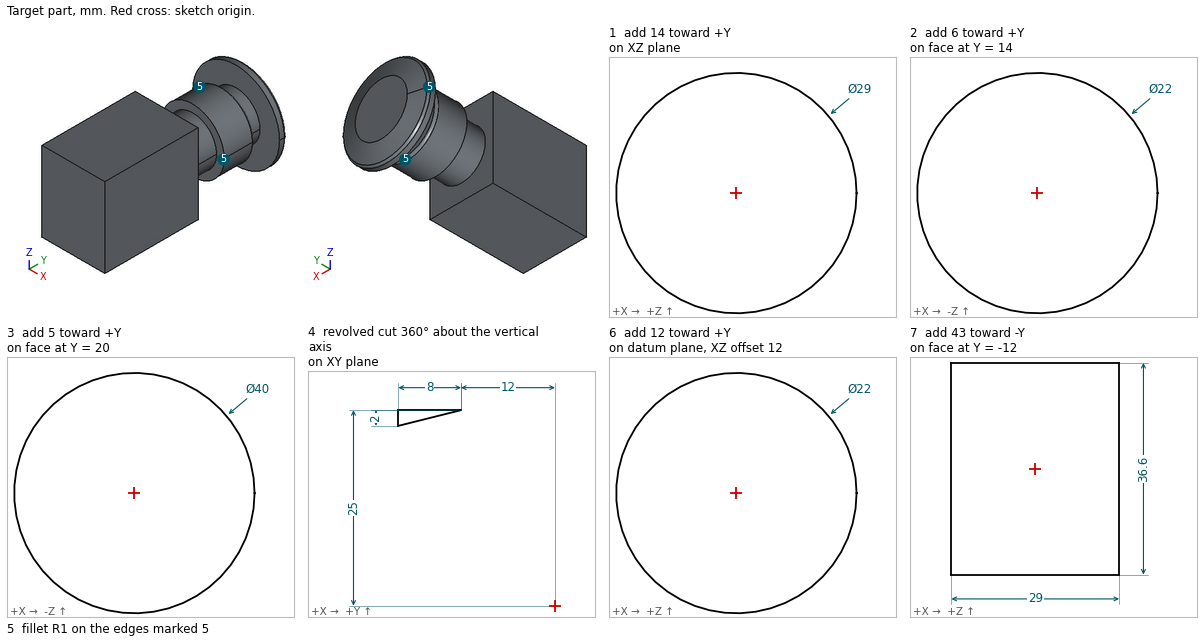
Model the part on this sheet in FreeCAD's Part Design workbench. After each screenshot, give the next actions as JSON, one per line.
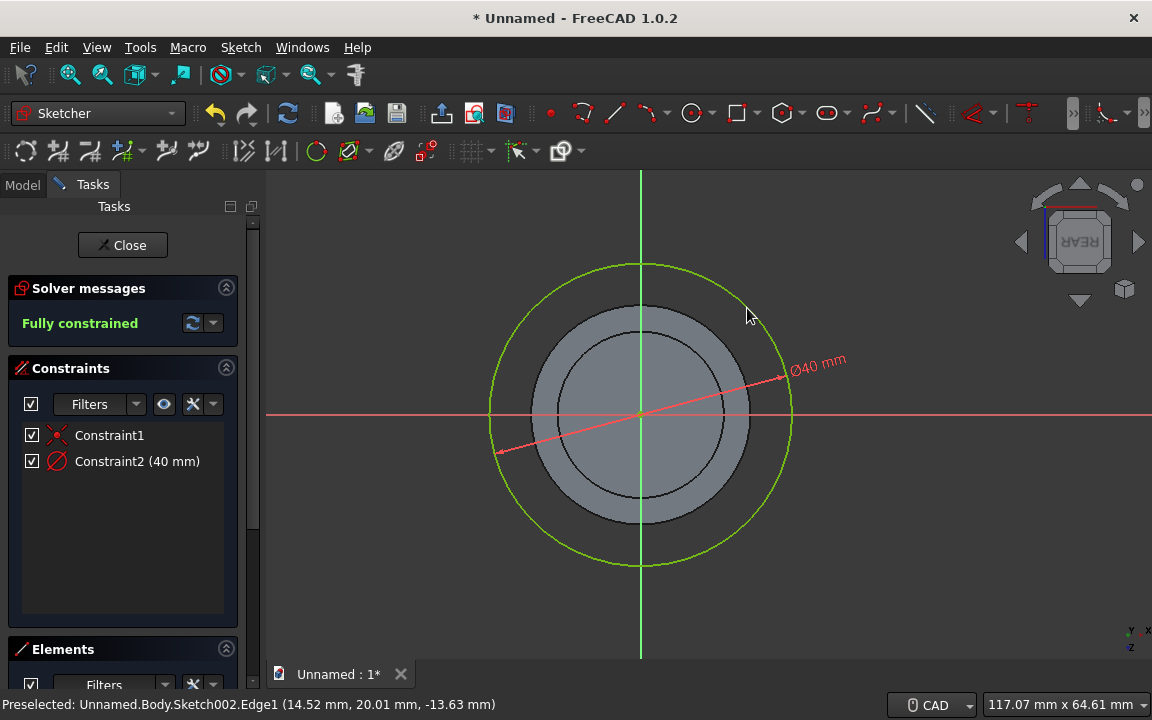
{"action": "left_click", "coordinate": [123, 245]}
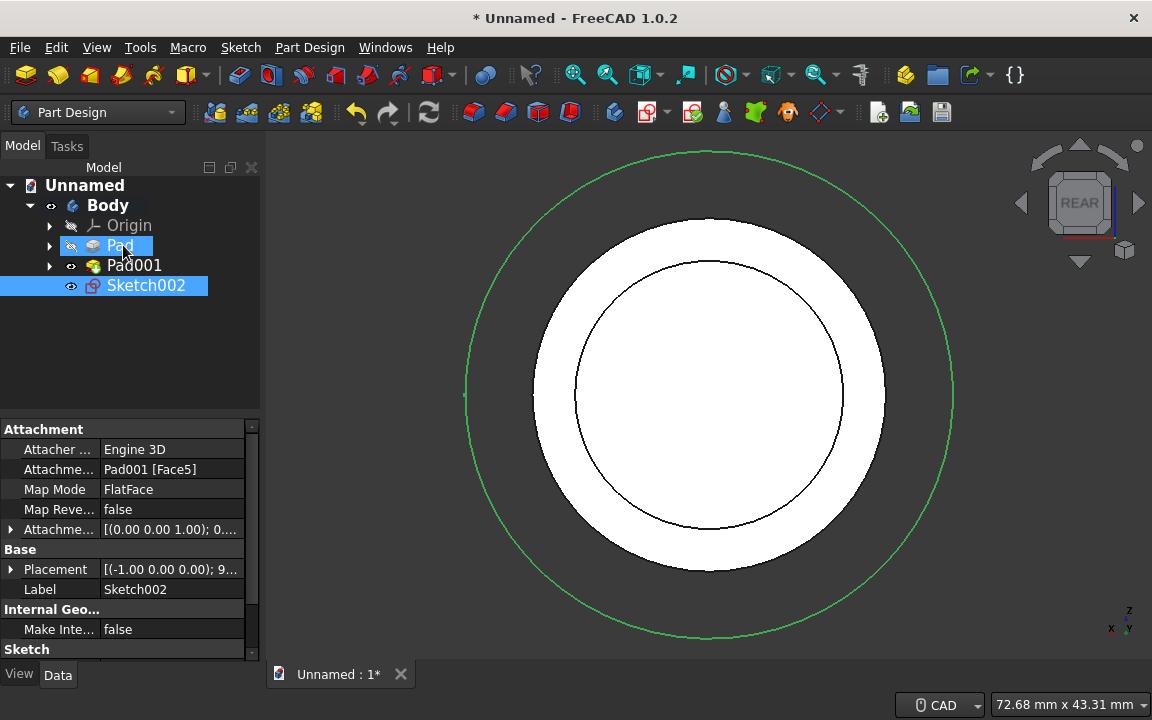
{"action": "left_click", "coordinate": [26, 76]}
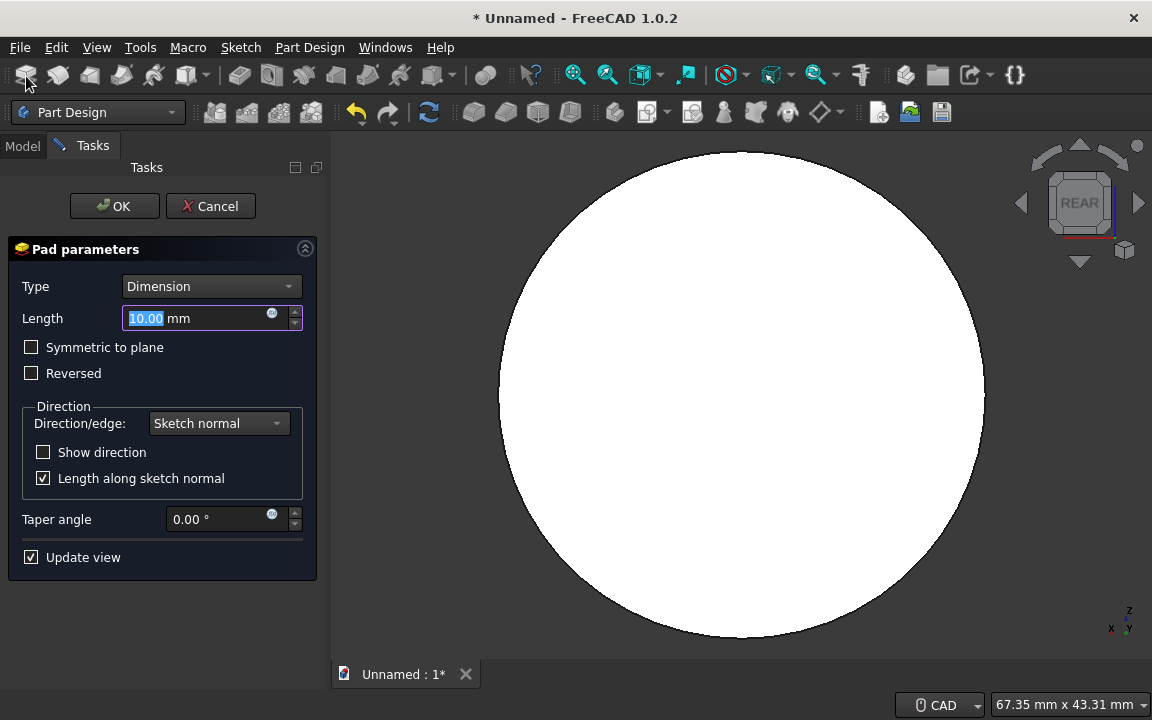
{"action": "type", "text": "5"}
{"action": "key", "text": "Tab"}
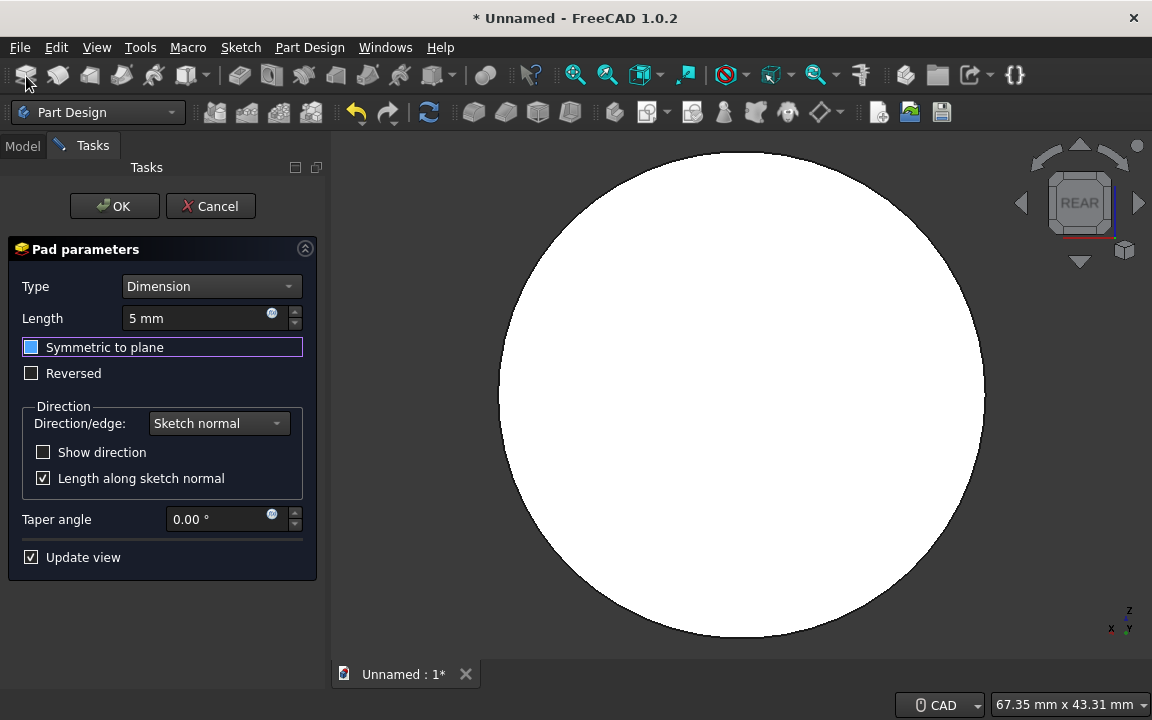
{"action": "left_click", "coordinate": [115, 206]}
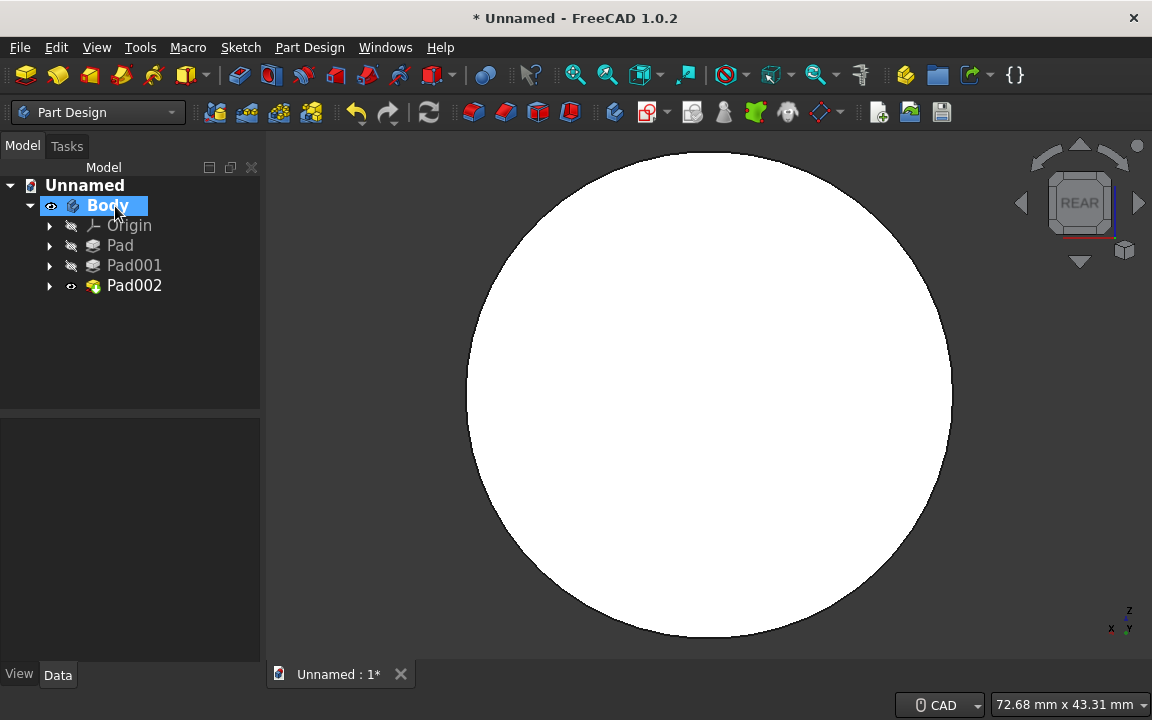
{"action": "left_click", "coordinate": [648, 112]}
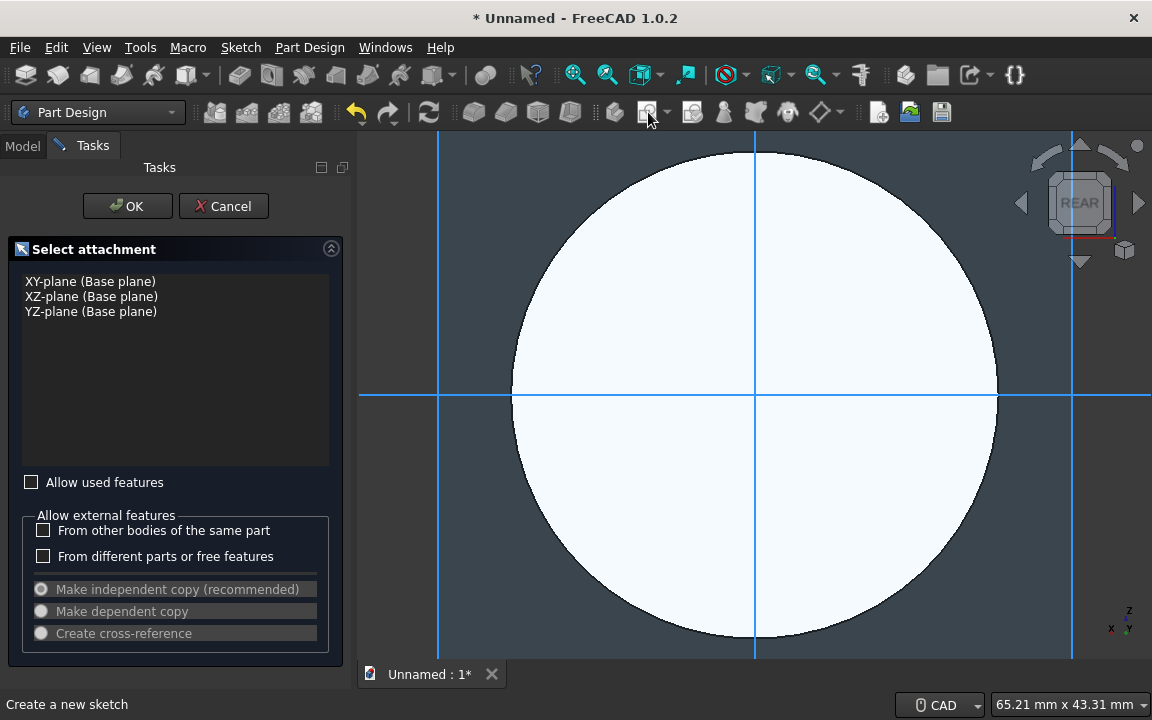
{"action": "left_click", "coordinate": [82, 282]}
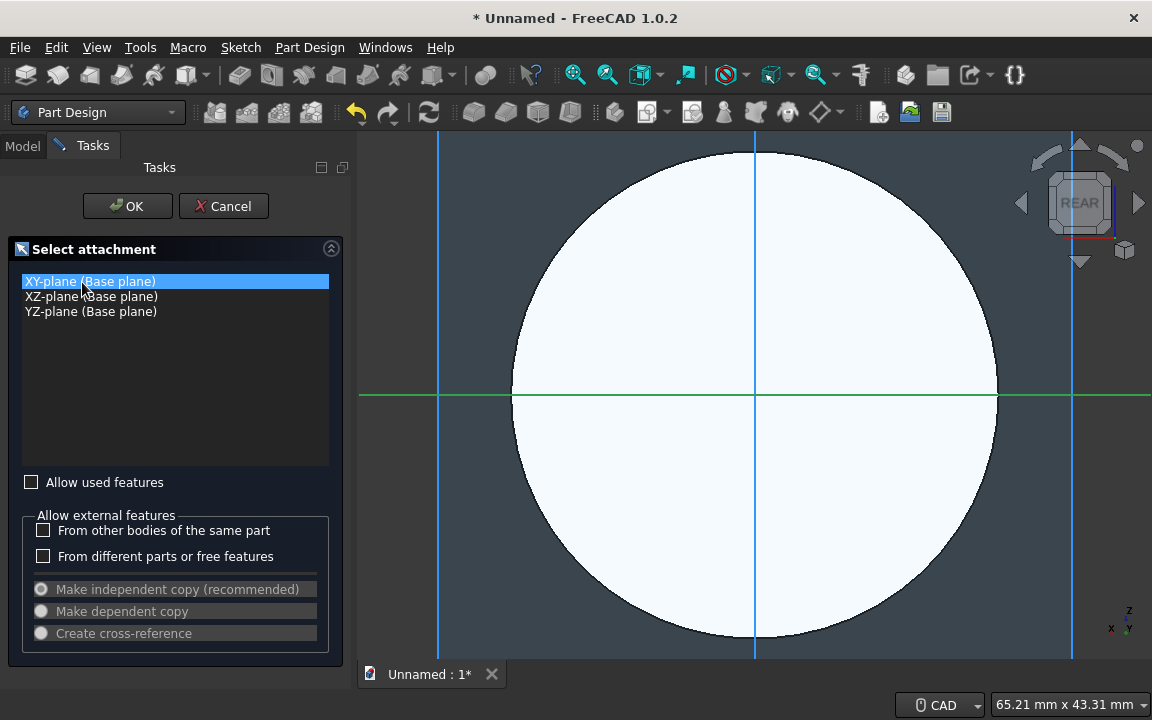
{"action": "left_click", "coordinate": [128, 206]}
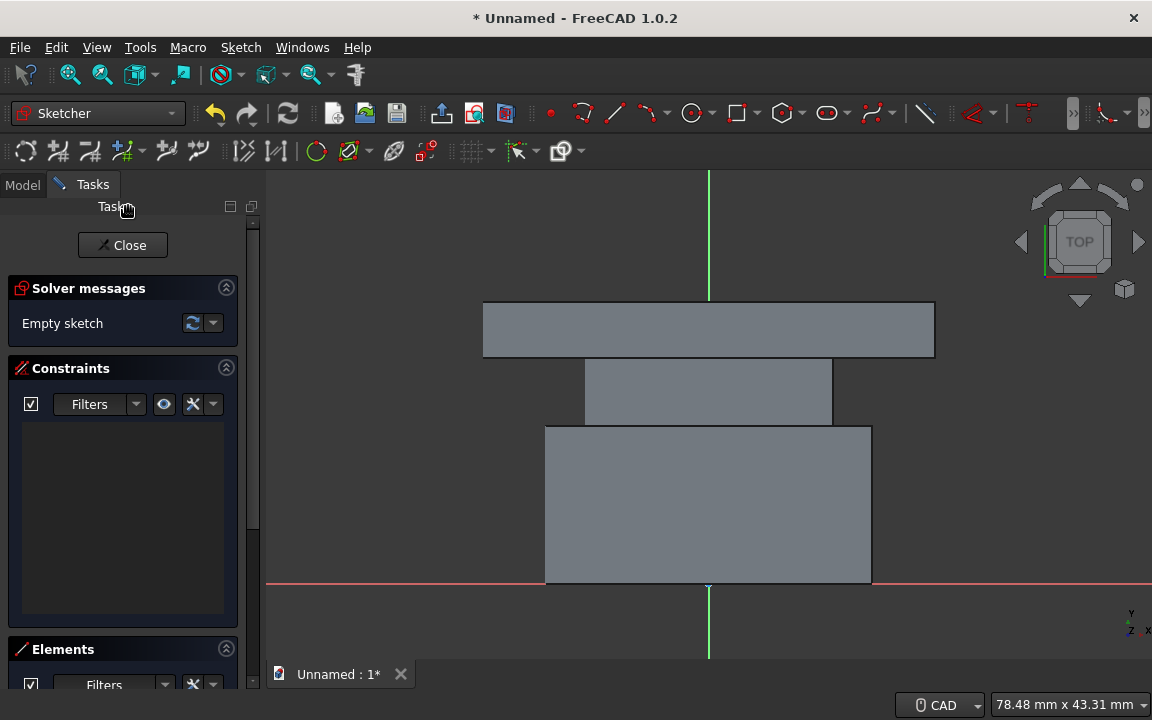
{"action": "key", "text": "q s"}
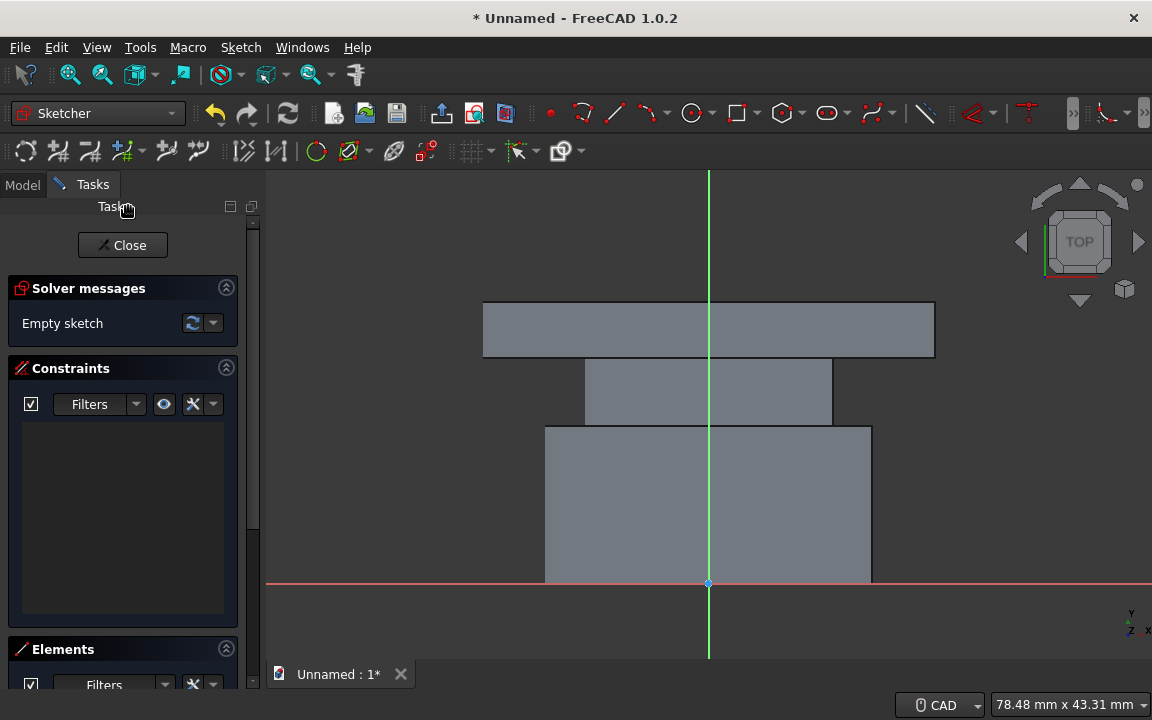
{"action": "scroll", "coordinate": [500, 287], "scroll_direction": "up", "scroll_amount": 8}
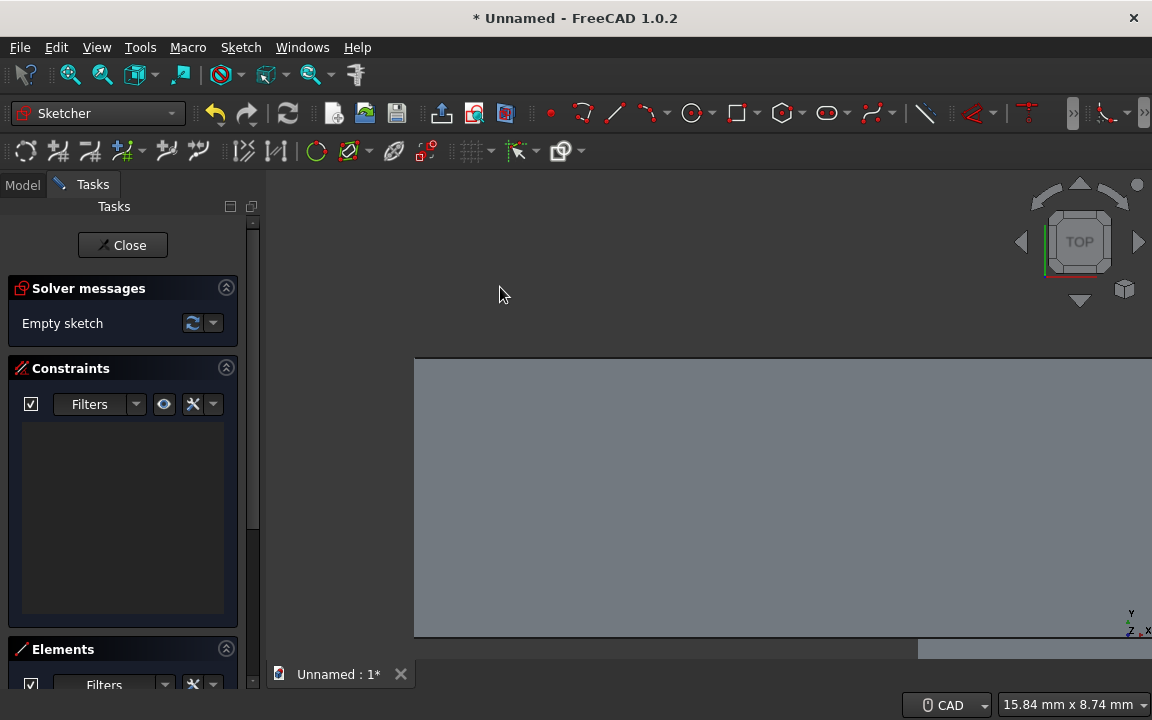
{"action": "key", "text": "g m"}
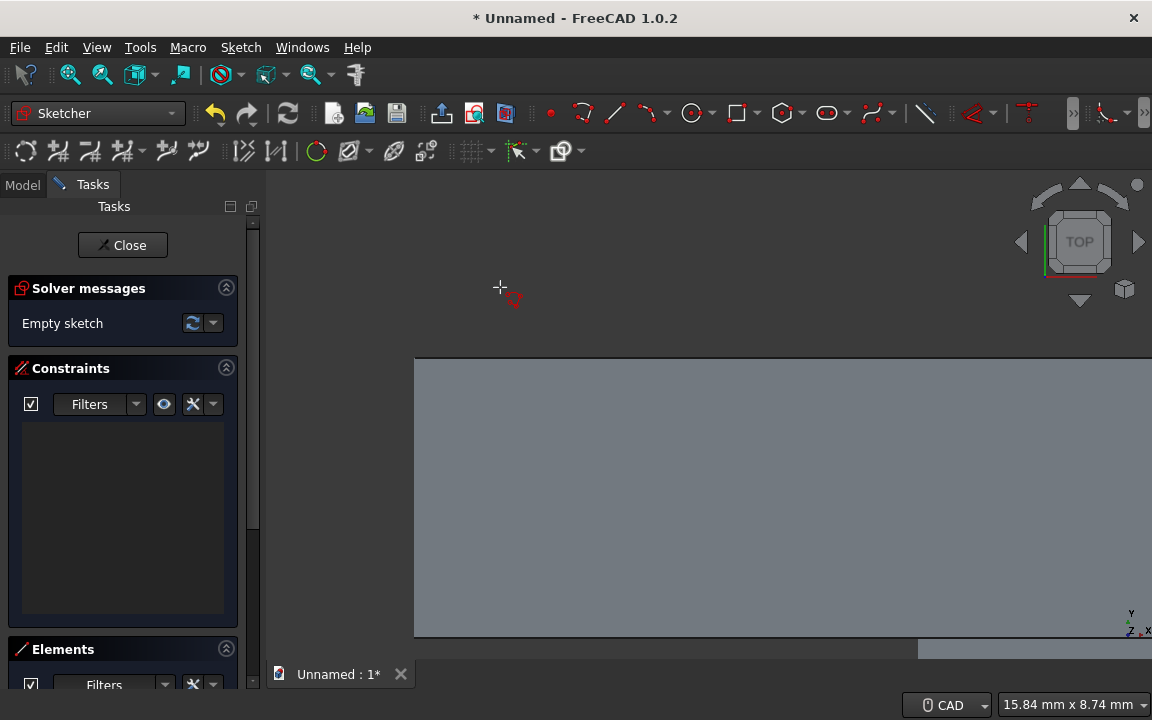
{"action": "left_click", "coordinate": [862, 358]}
{"action": "left_click", "coordinate": [414, 358]}
{"action": "left_click", "coordinate": [414, 470]}
{"action": "left_click", "coordinate": [862, 359]}
{"action": "key", "text": "Escape"}
{"action": "key", "text": "Escape"}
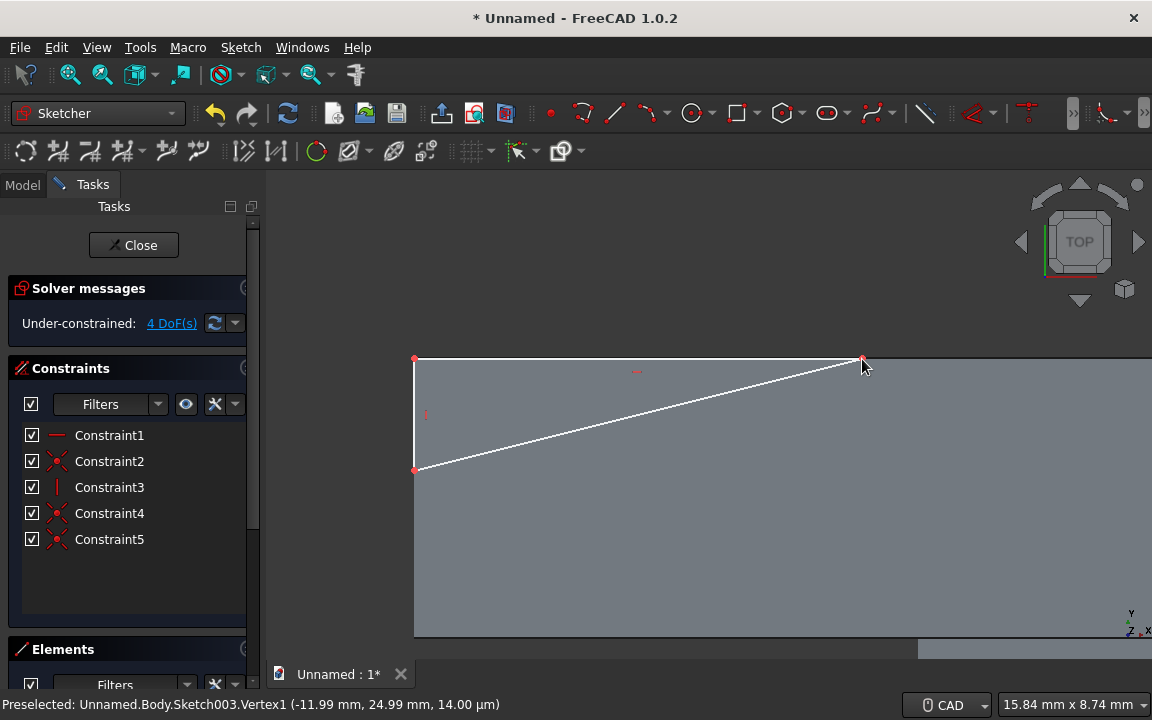
{"action": "left_click", "coordinate": [728, 359]}